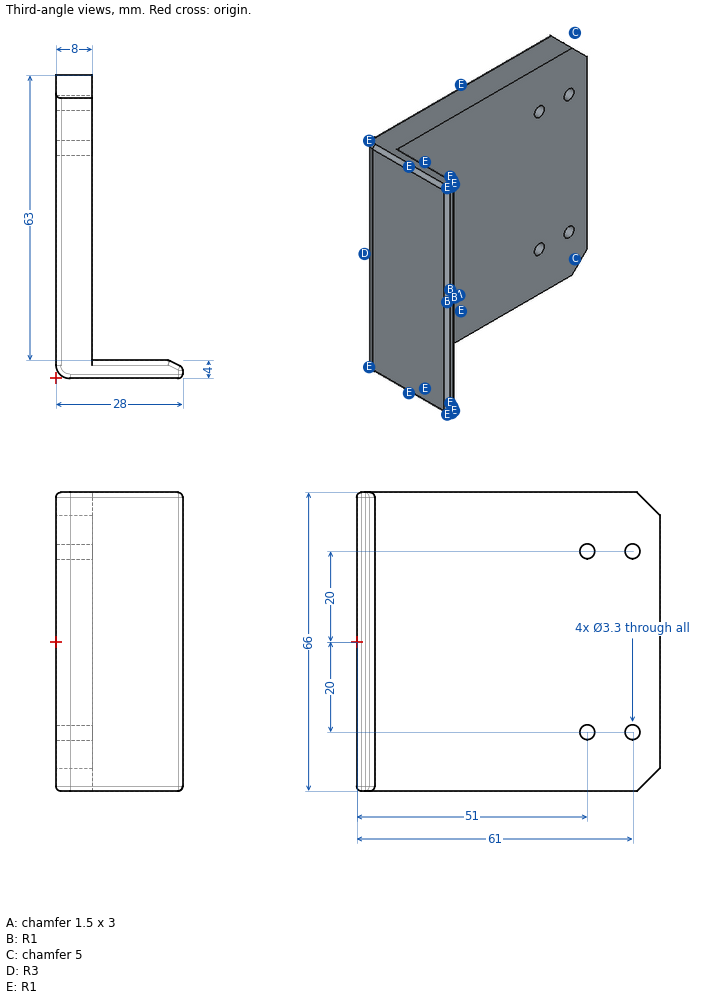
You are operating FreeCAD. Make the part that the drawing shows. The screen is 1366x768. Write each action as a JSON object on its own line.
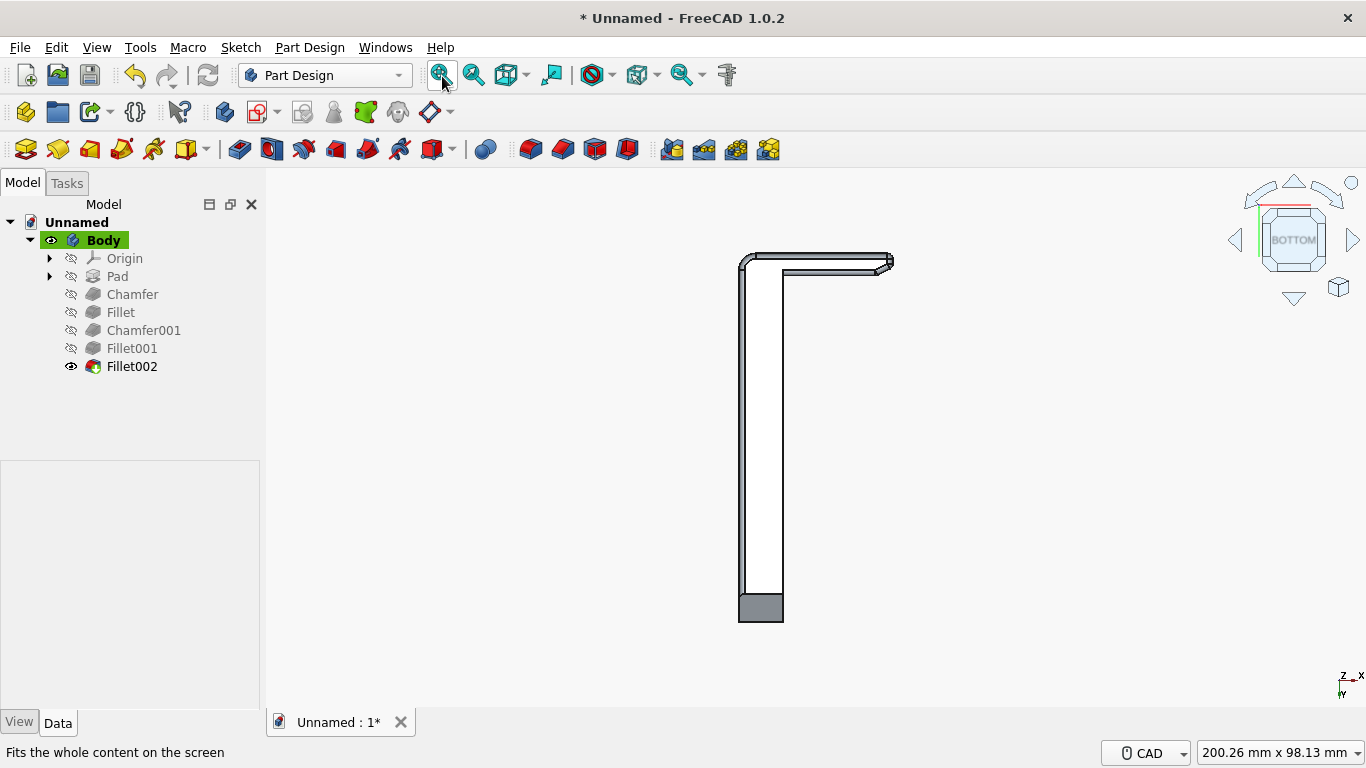
{"action": "left_click", "coordinate": [258, 112]}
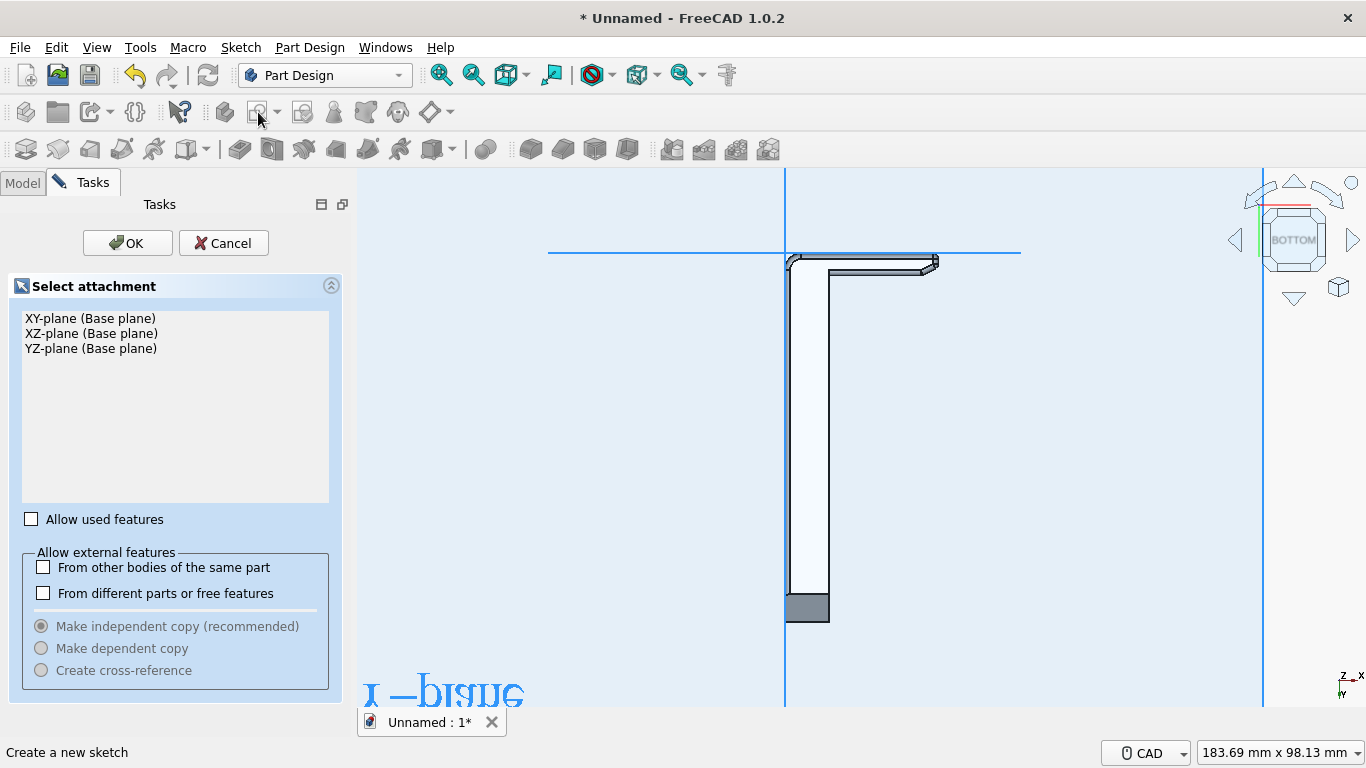
{"action": "left_click", "coordinate": [82, 348]}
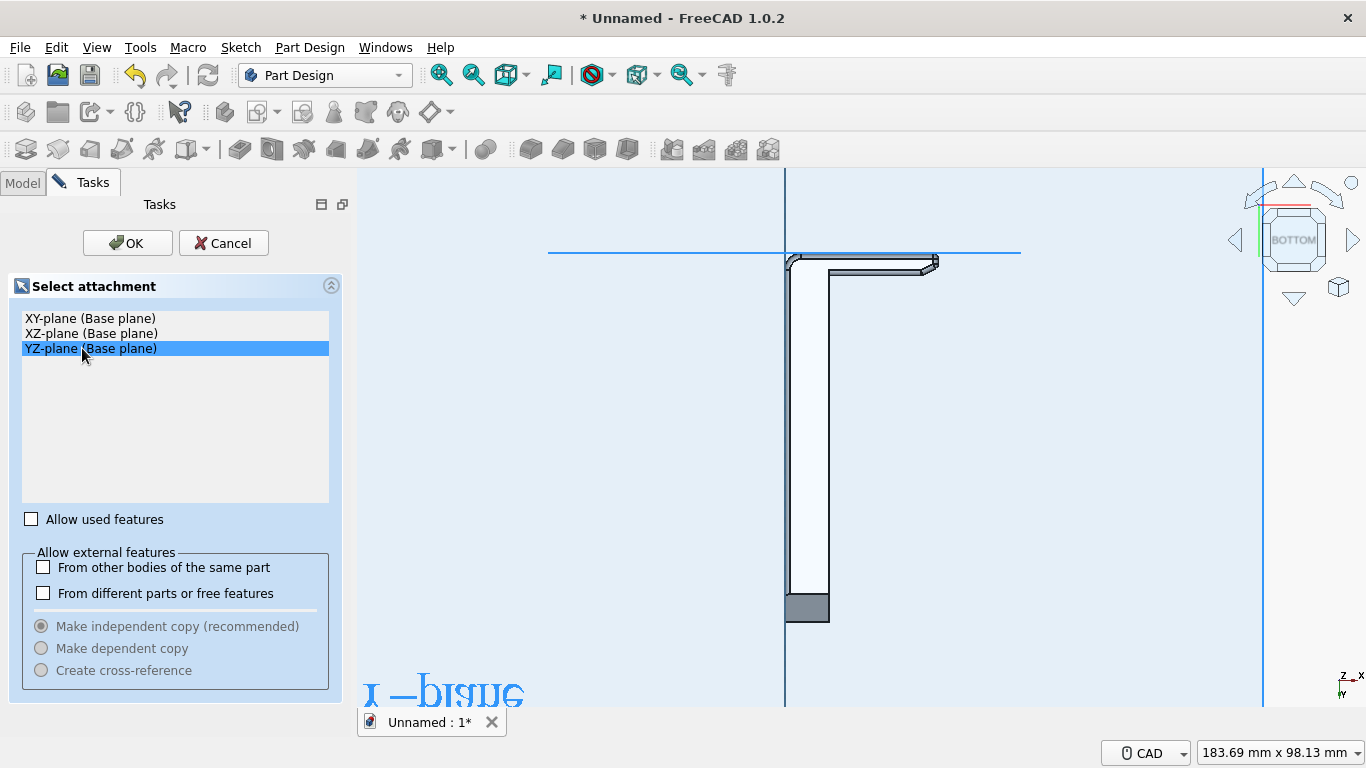
{"action": "left_click", "coordinate": [128, 243]}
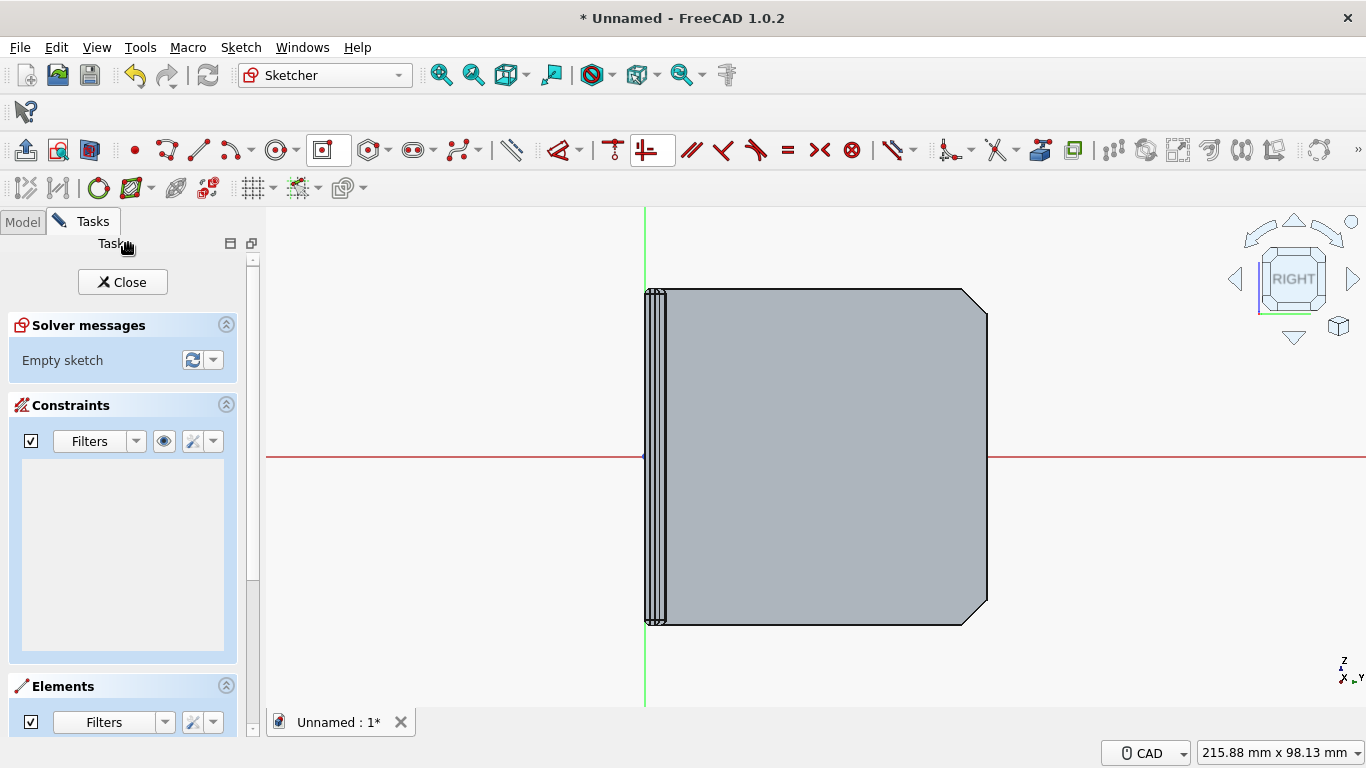
{"action": "key", "text": "q s"}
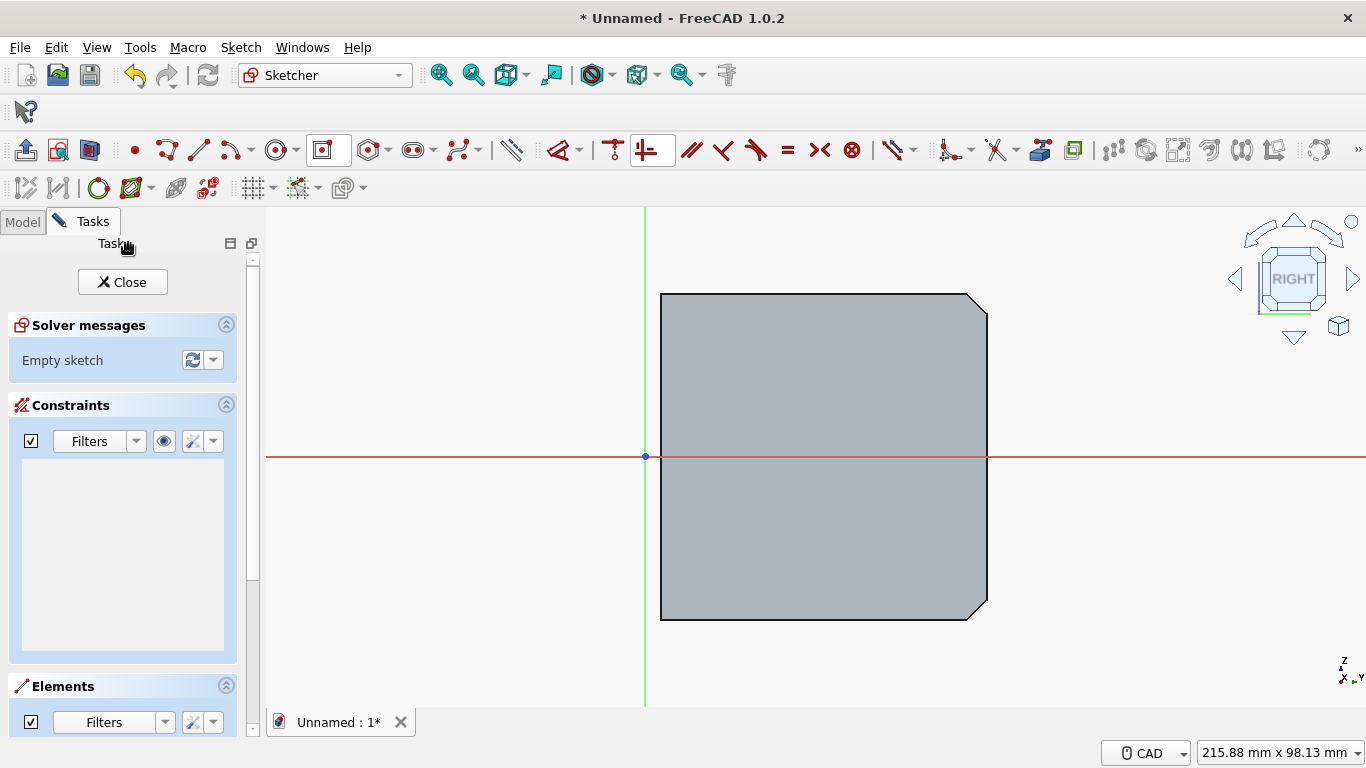
{"action": "scroll", "coordinate": [922, 457], "scroll_direction": "up", "scroll_amount": 2}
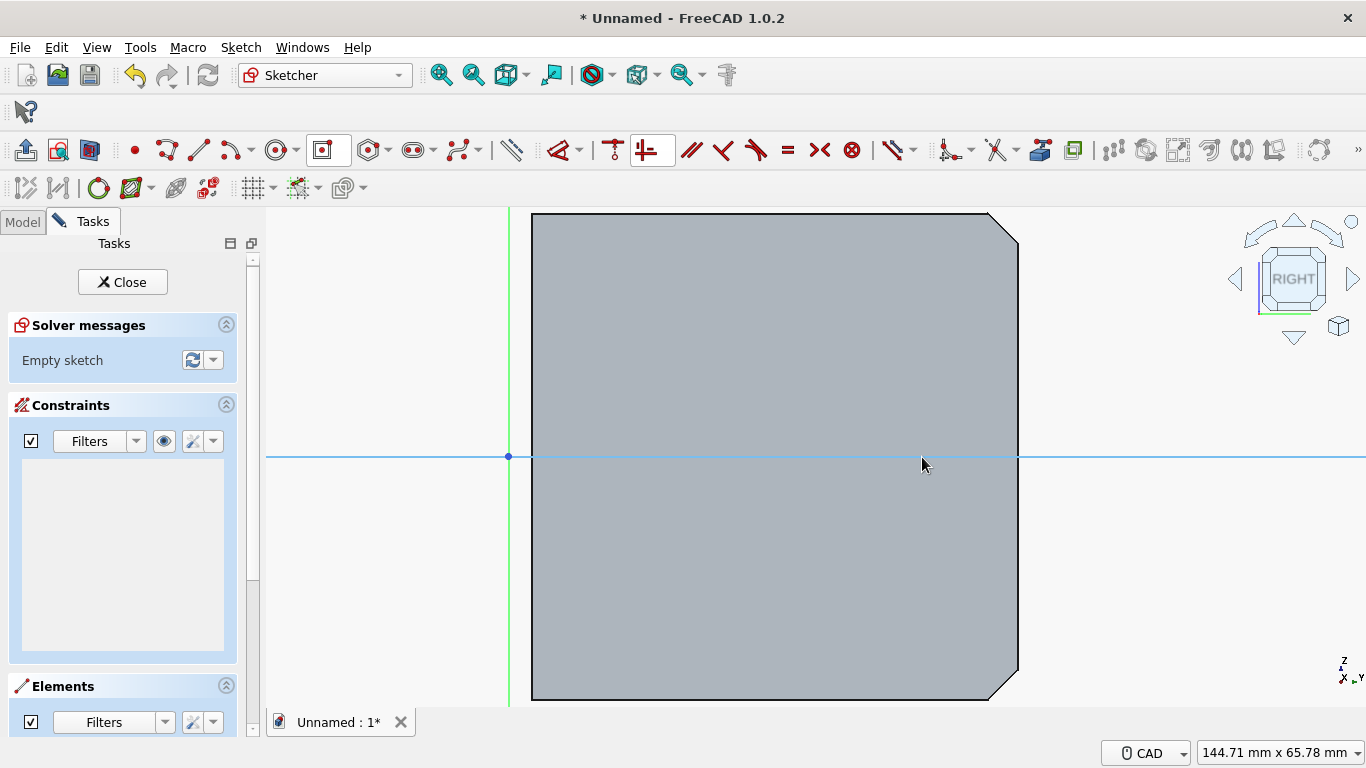
{"action": "left_click", "coordinate": [276, 150]}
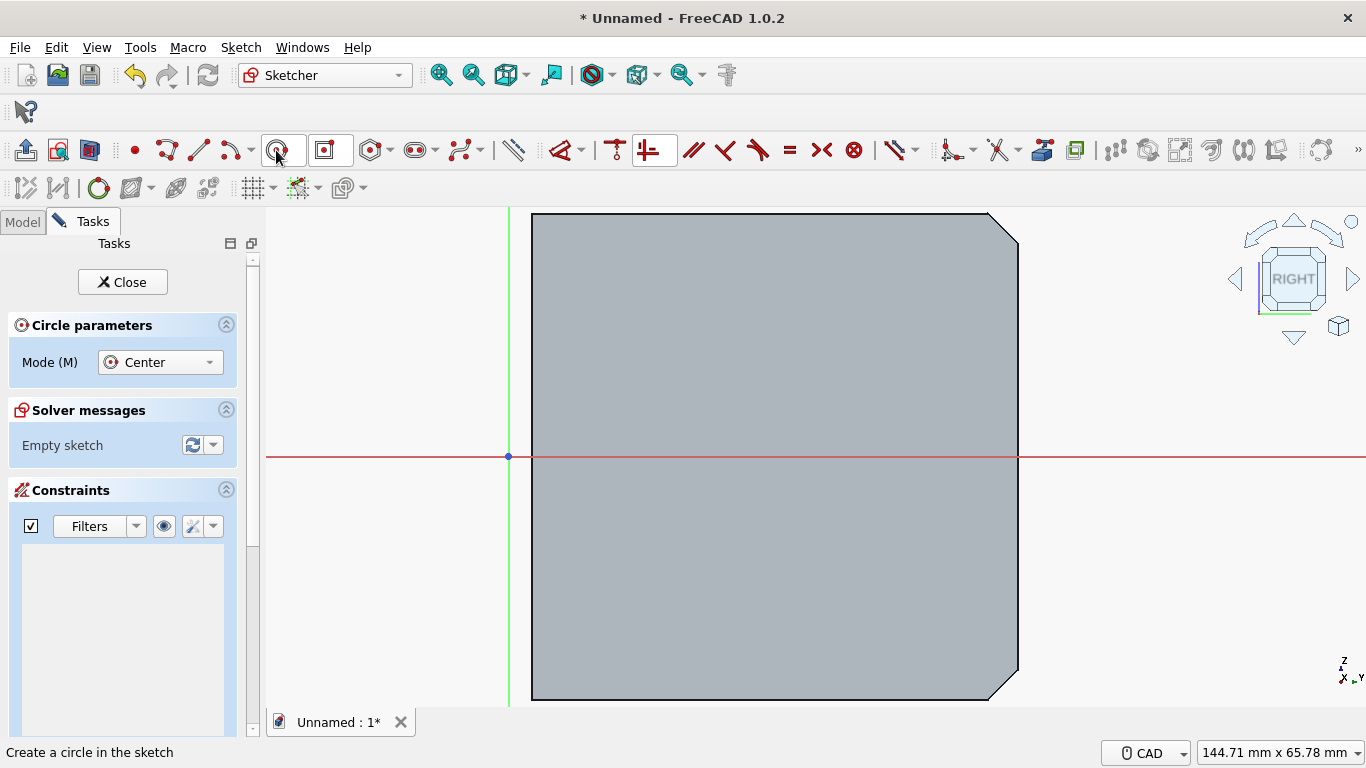
{"action": "scroll", "coordinate": [973, 609], "scroll_direction": "up", "scroll_amount": 3}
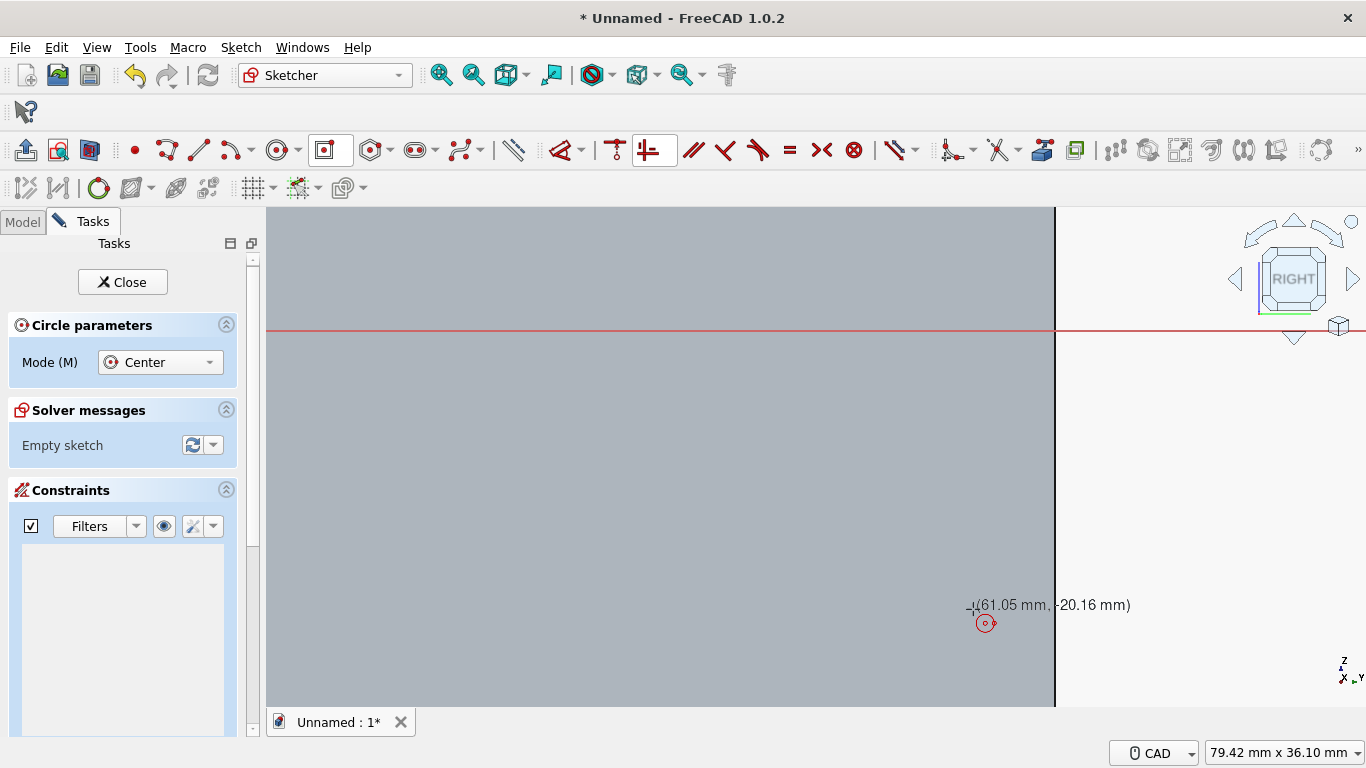
{"action": "left_click", "coordinate": [972, 608]}
{"action": "mouse_move", "coordinate": [988, 592]}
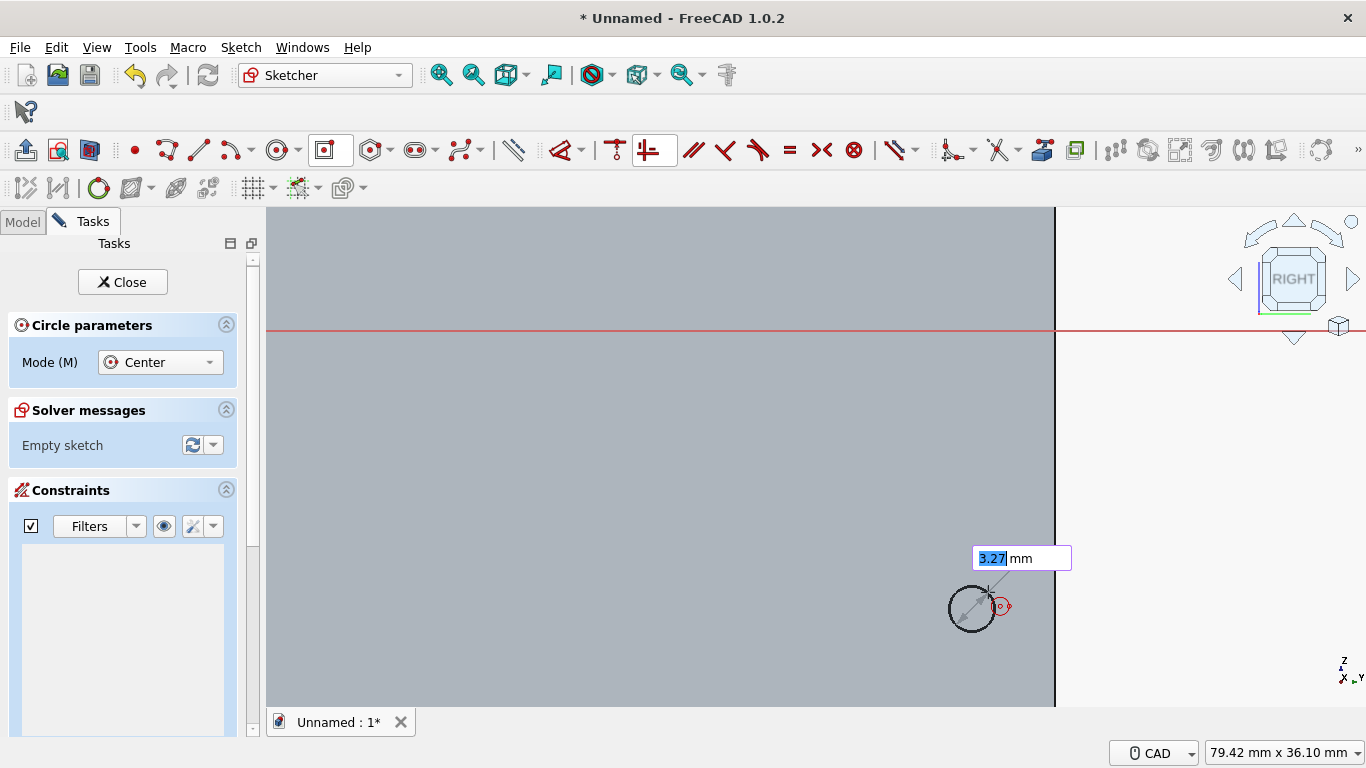
{"action": "type", "text": "3.3"}
{"action": "key", "text": "Return"}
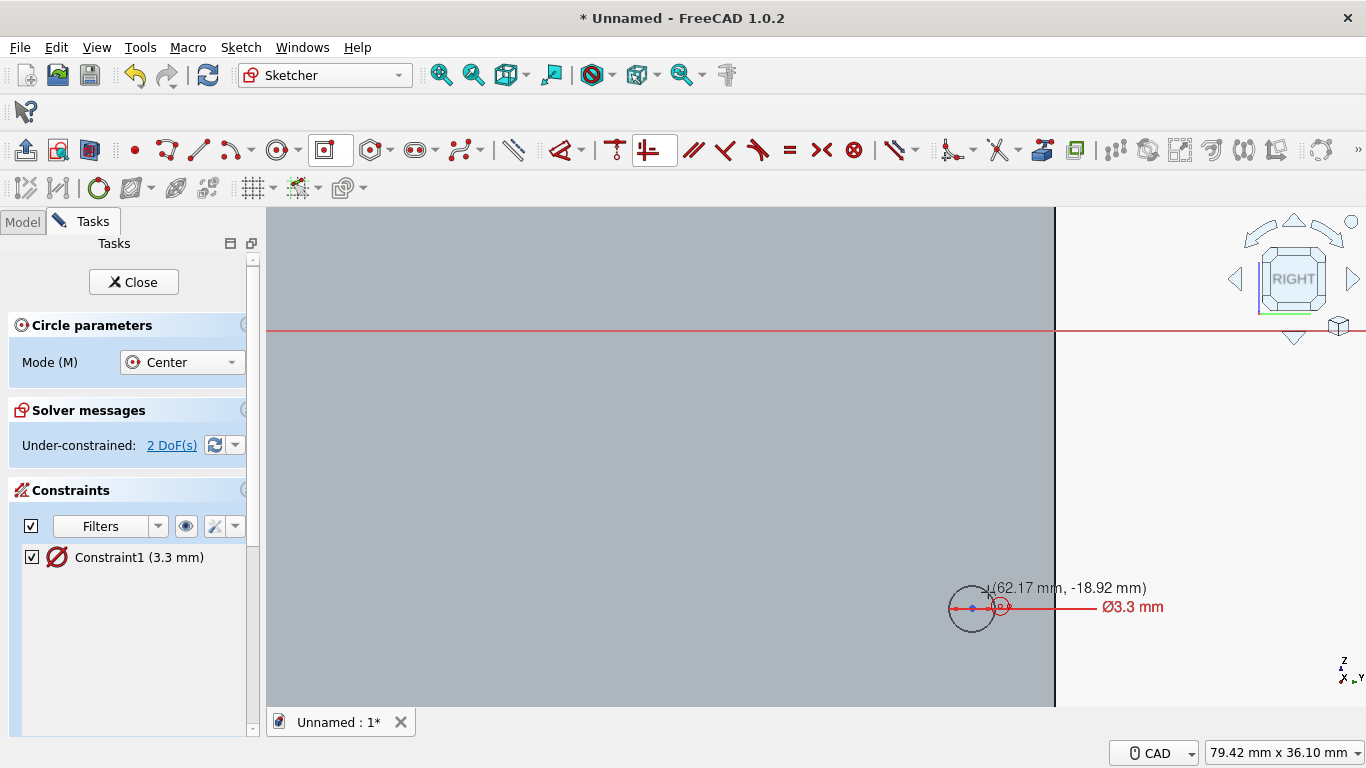
{"action": "scroll", "coordinate": [975, 610], "scroll_direction": "down", "scroll_amount": 3}